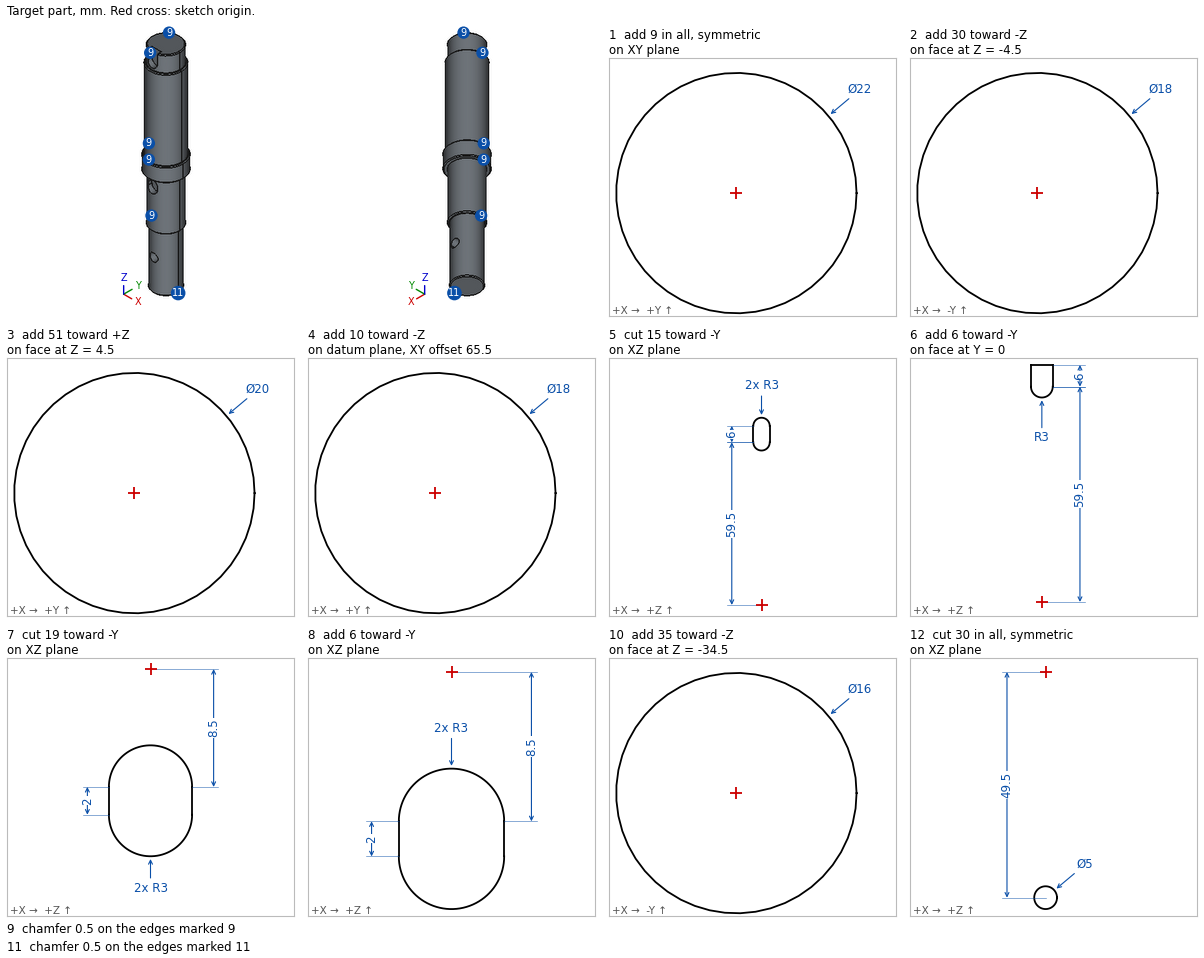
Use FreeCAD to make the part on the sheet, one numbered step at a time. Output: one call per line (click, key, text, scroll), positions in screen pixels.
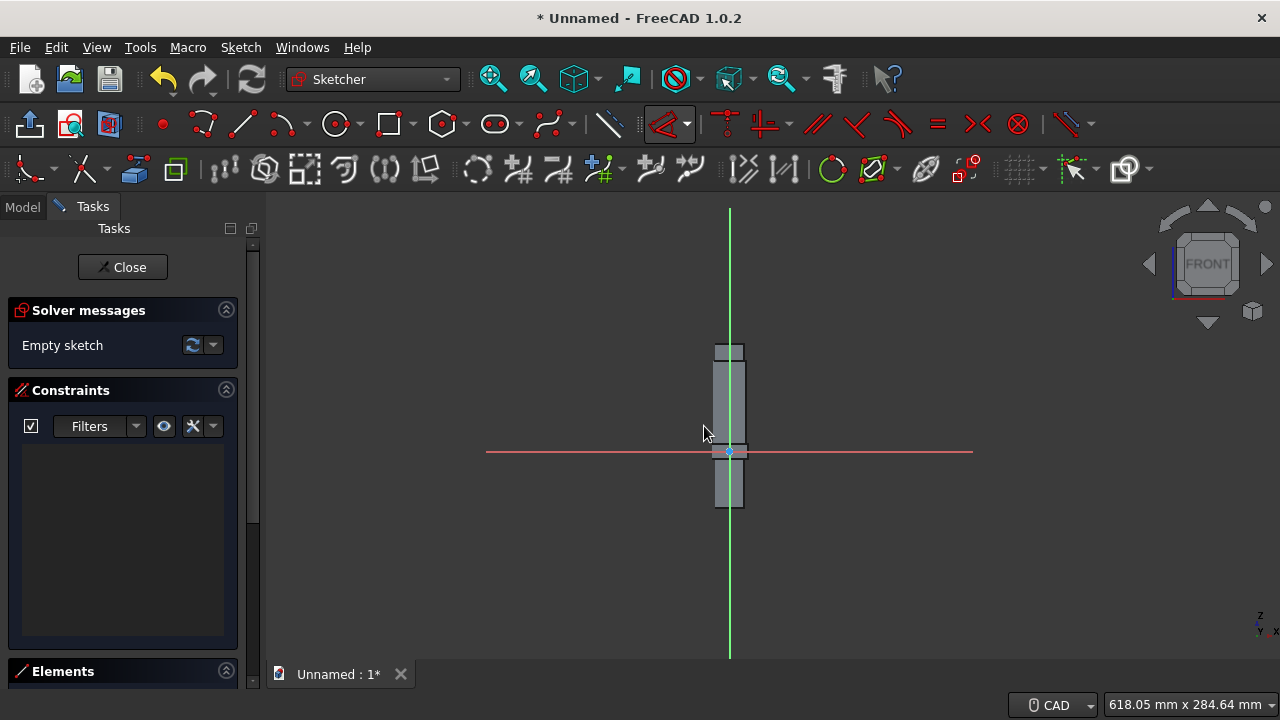
scroll(732, 343, up, 13)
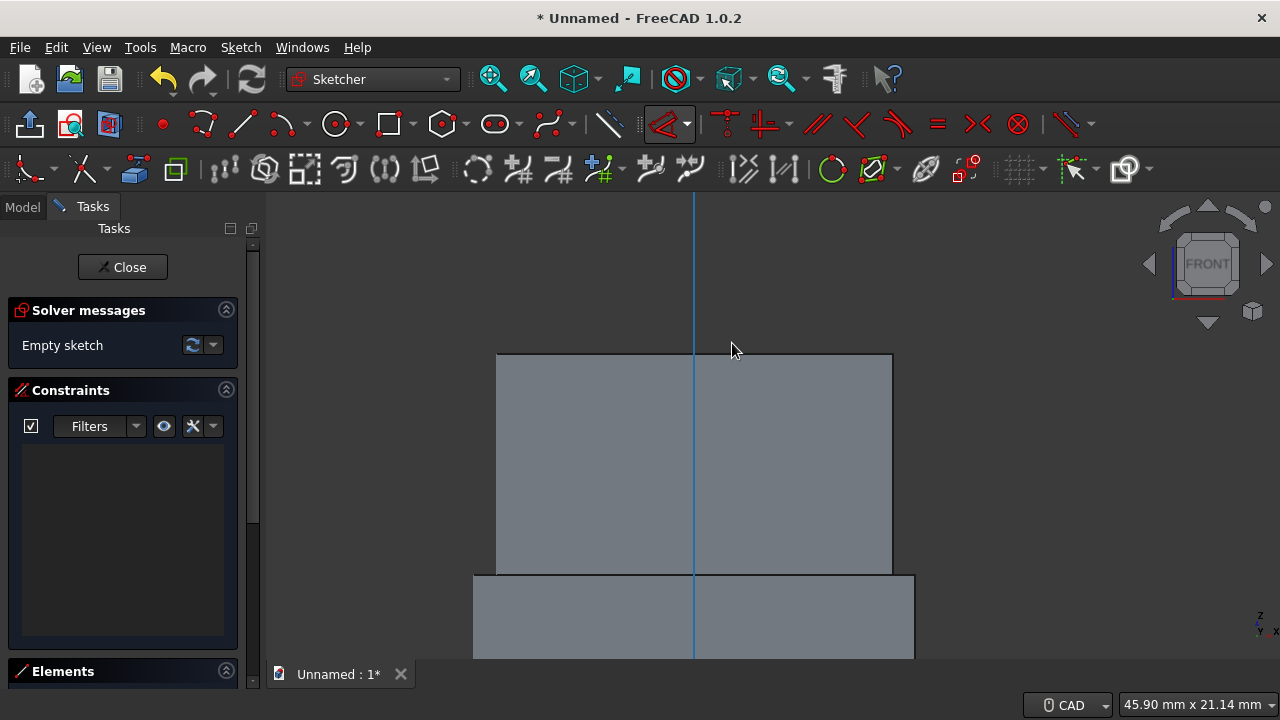
click(496, 124)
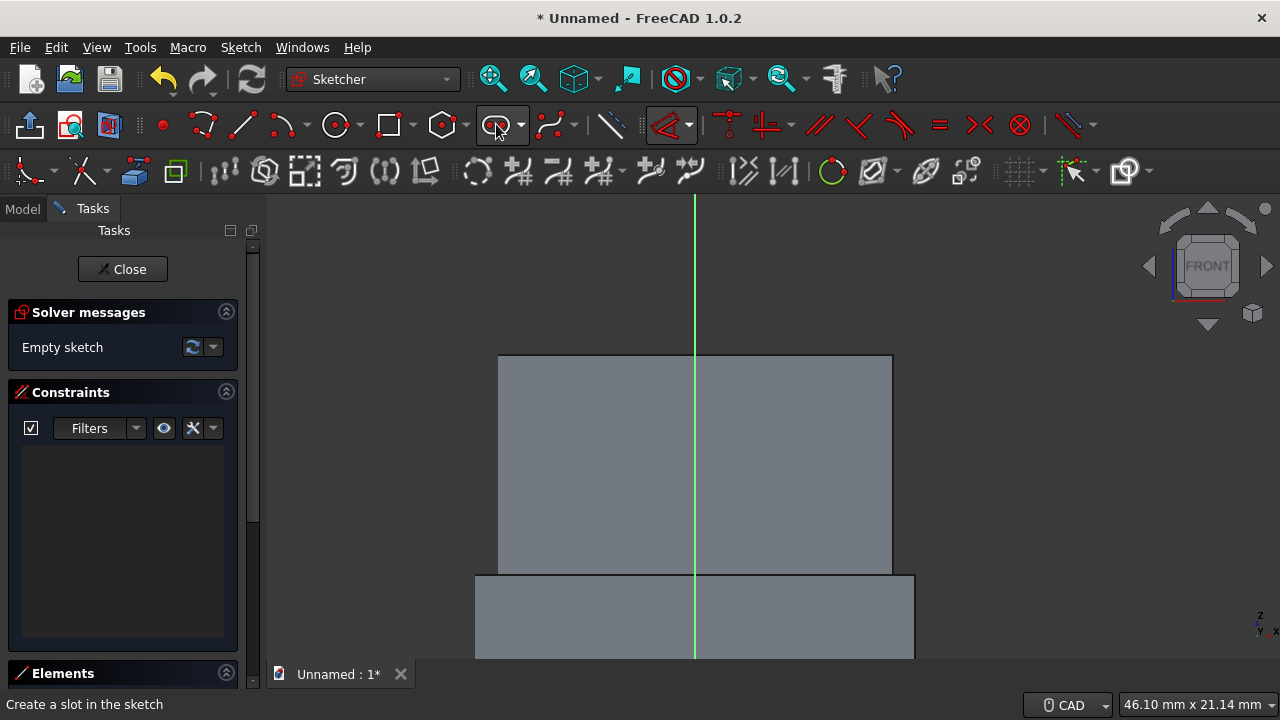
click(695, 487)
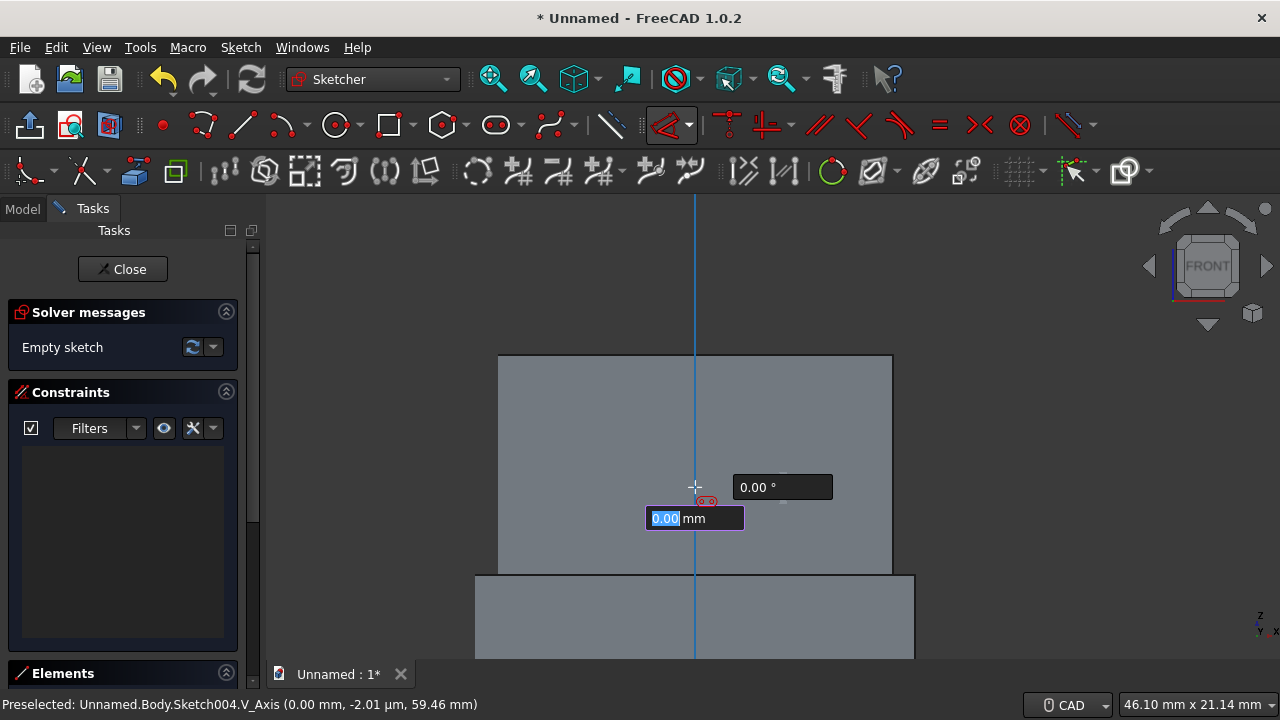
click(704, 355)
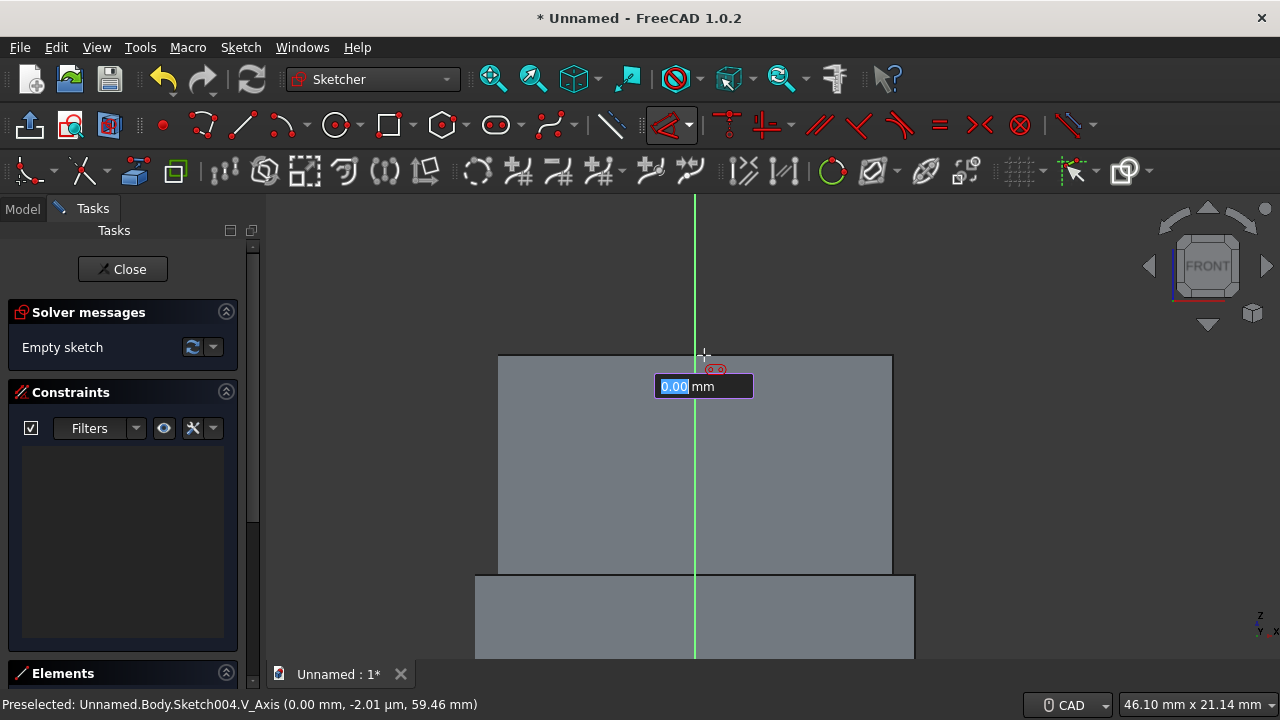
click(629, 421)
key(Escape)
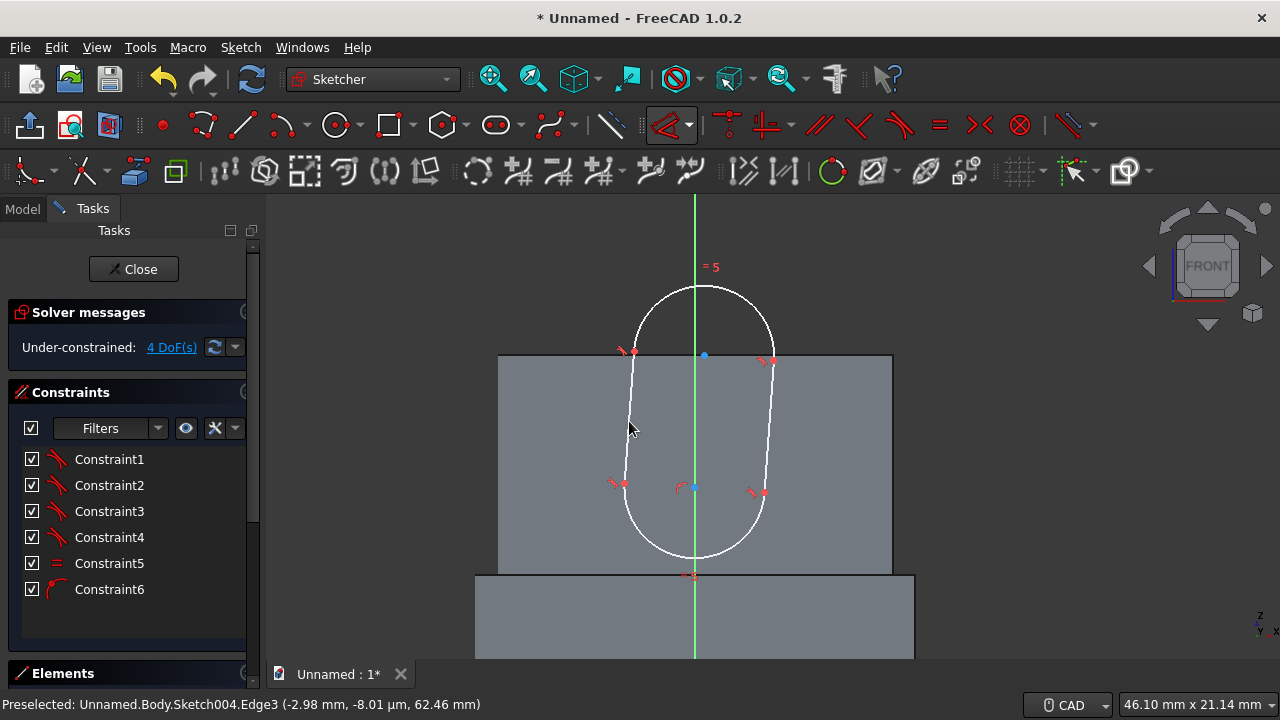
click(627, 443)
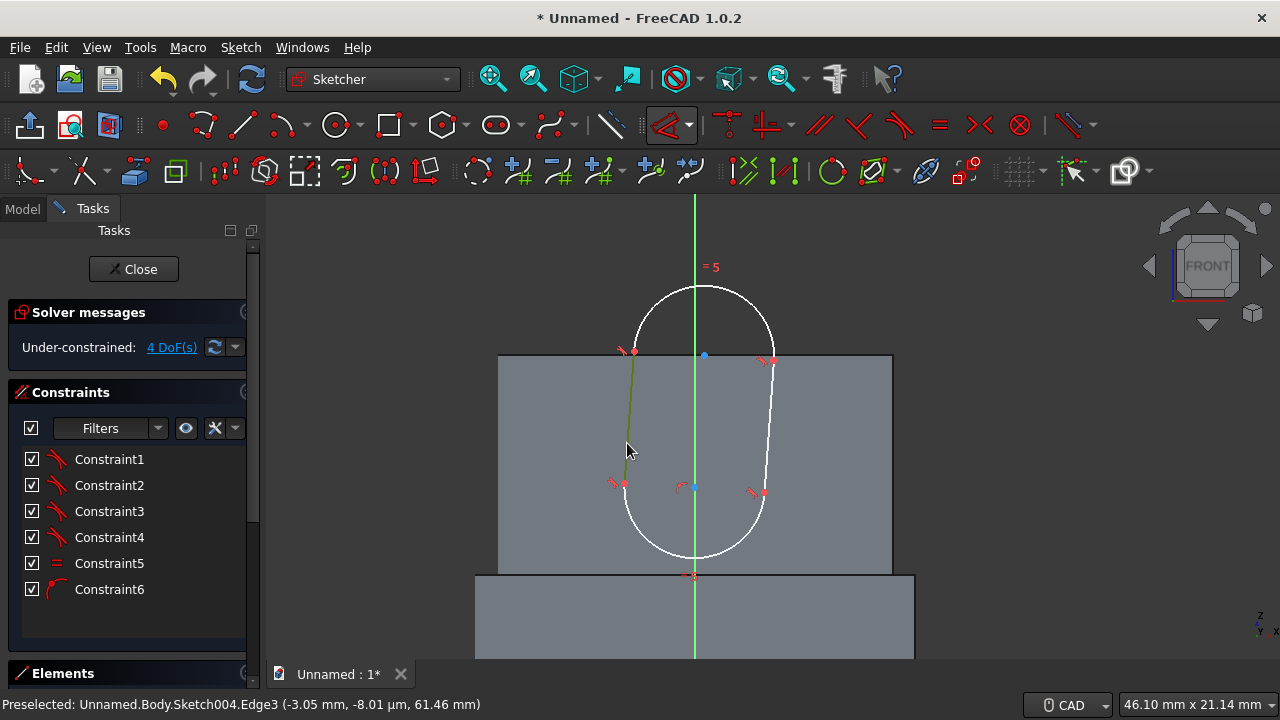
key(v)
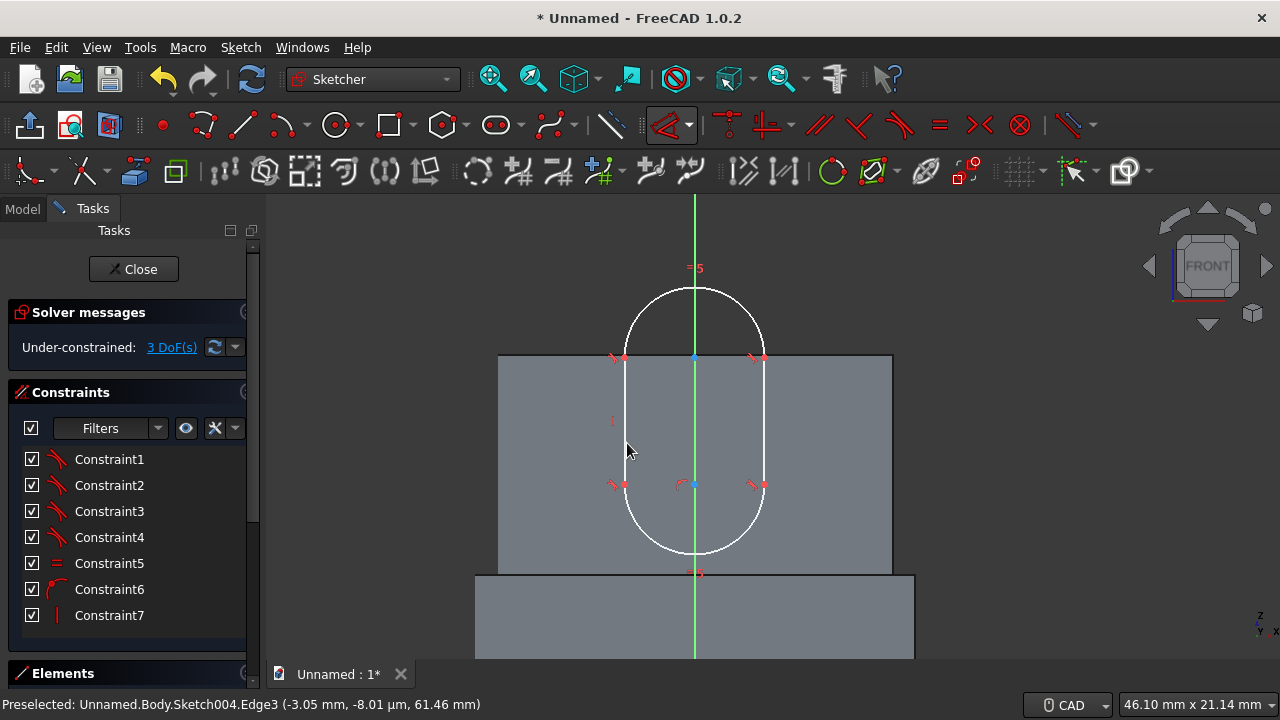
click(654, 541)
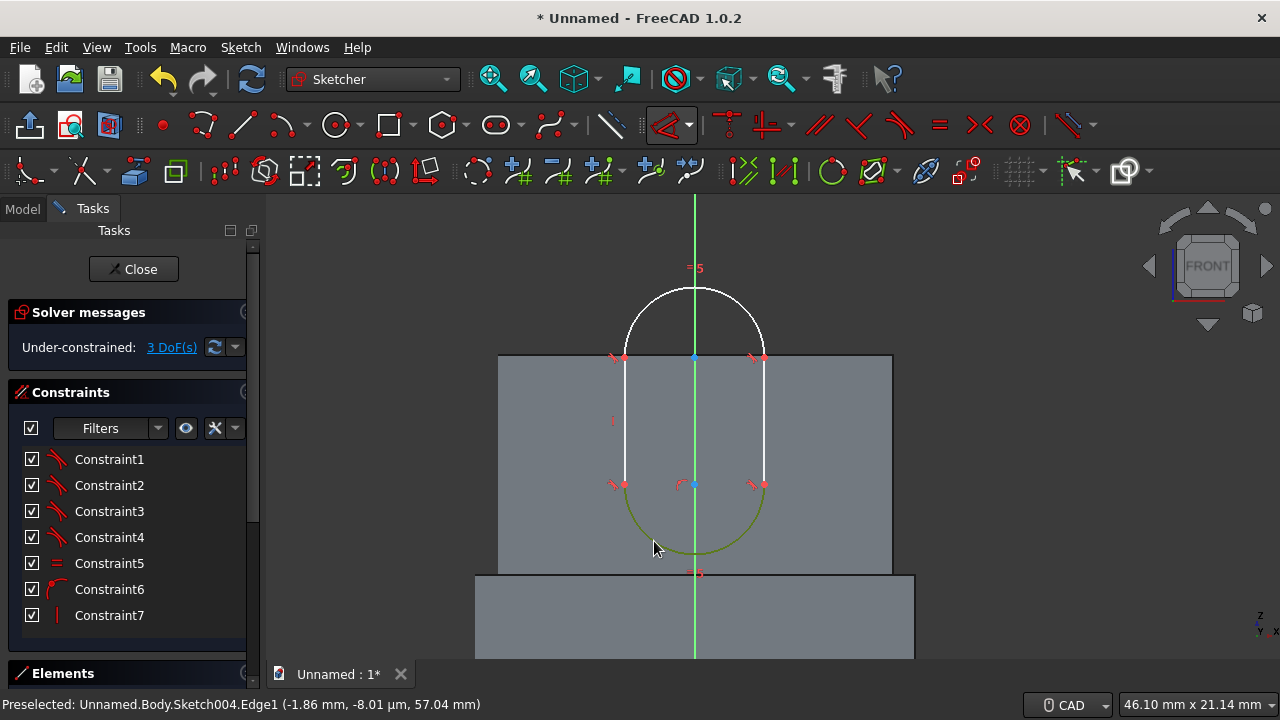
key(k)
key(r)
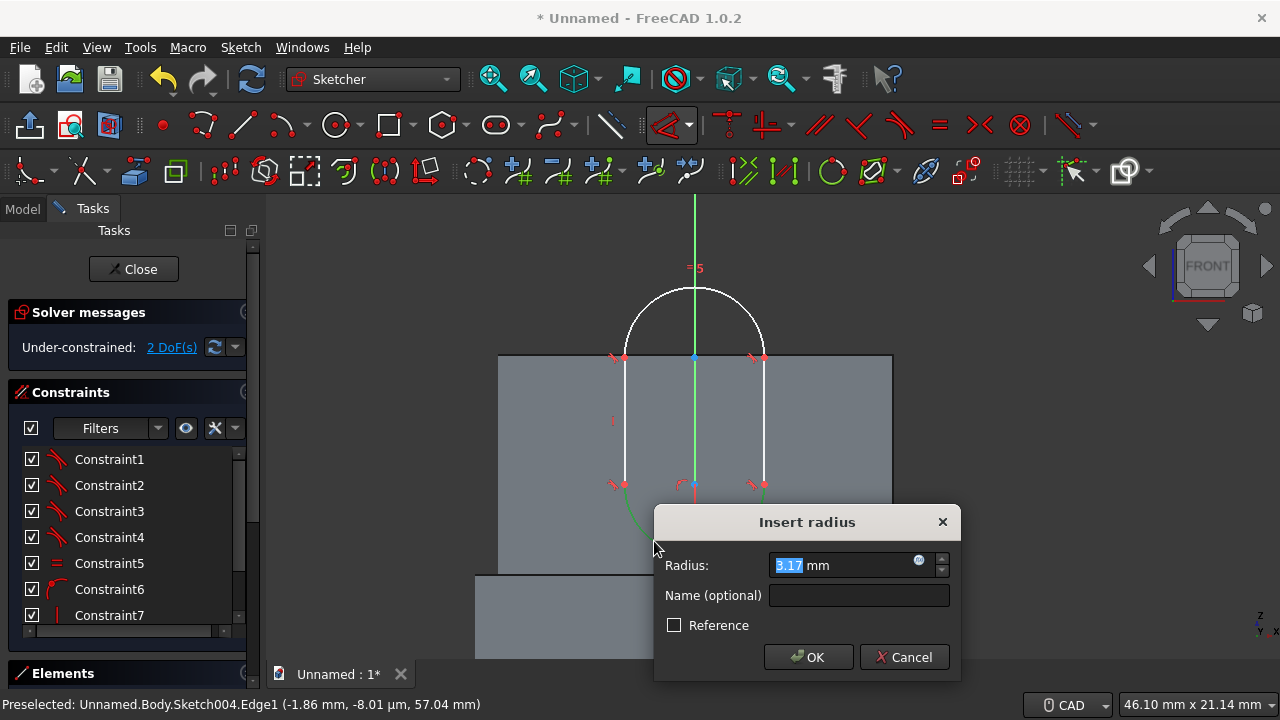
text(3)
key(Return)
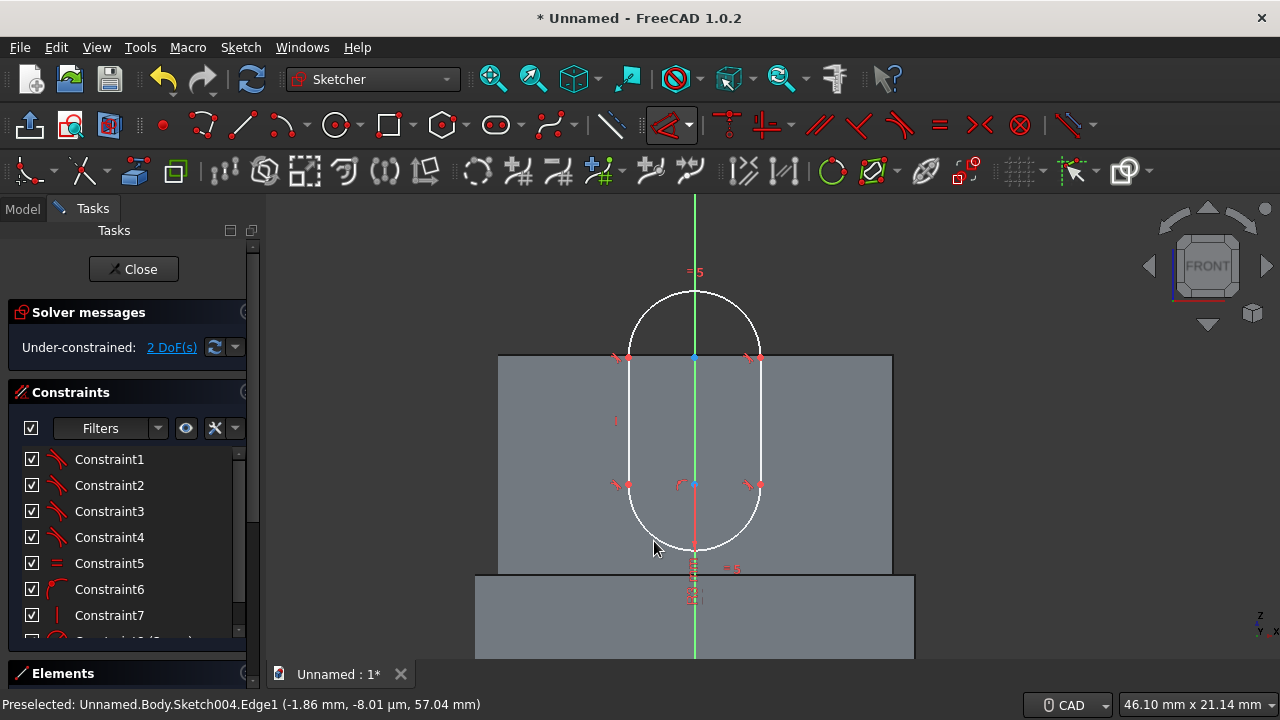
click(629, 446)